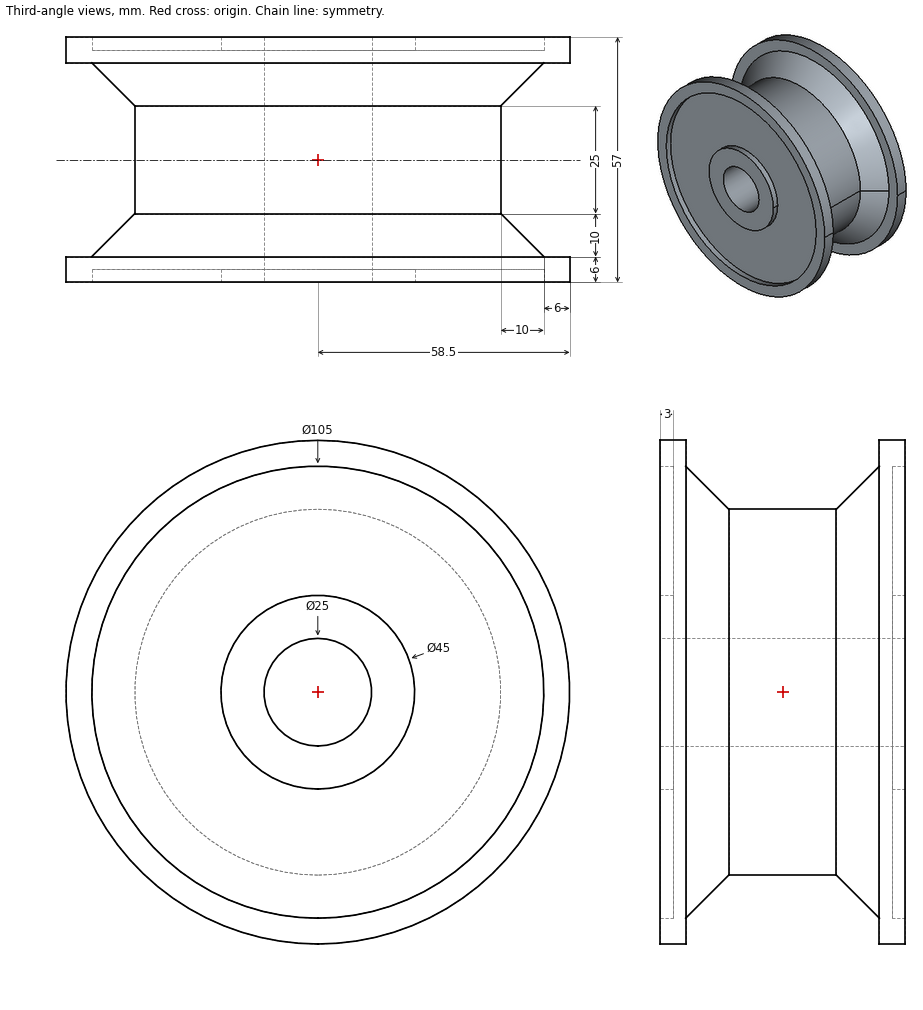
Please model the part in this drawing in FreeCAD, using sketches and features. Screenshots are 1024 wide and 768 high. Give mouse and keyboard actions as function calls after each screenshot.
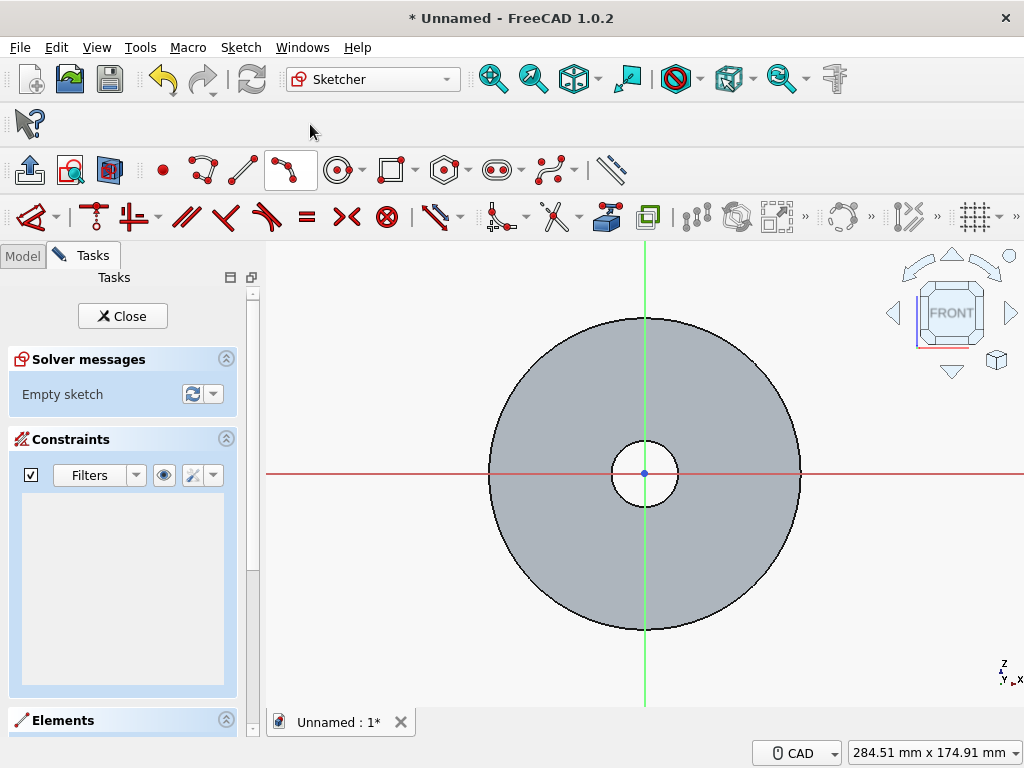
click(338, 170)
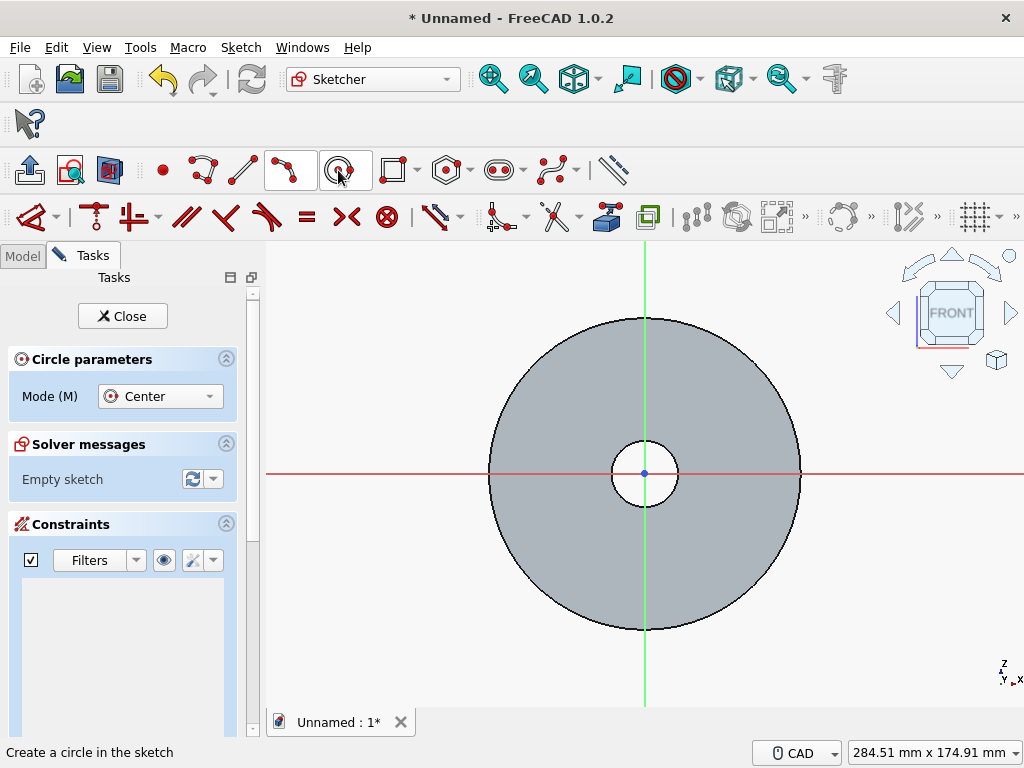
click(645, 474)
click(744, 375)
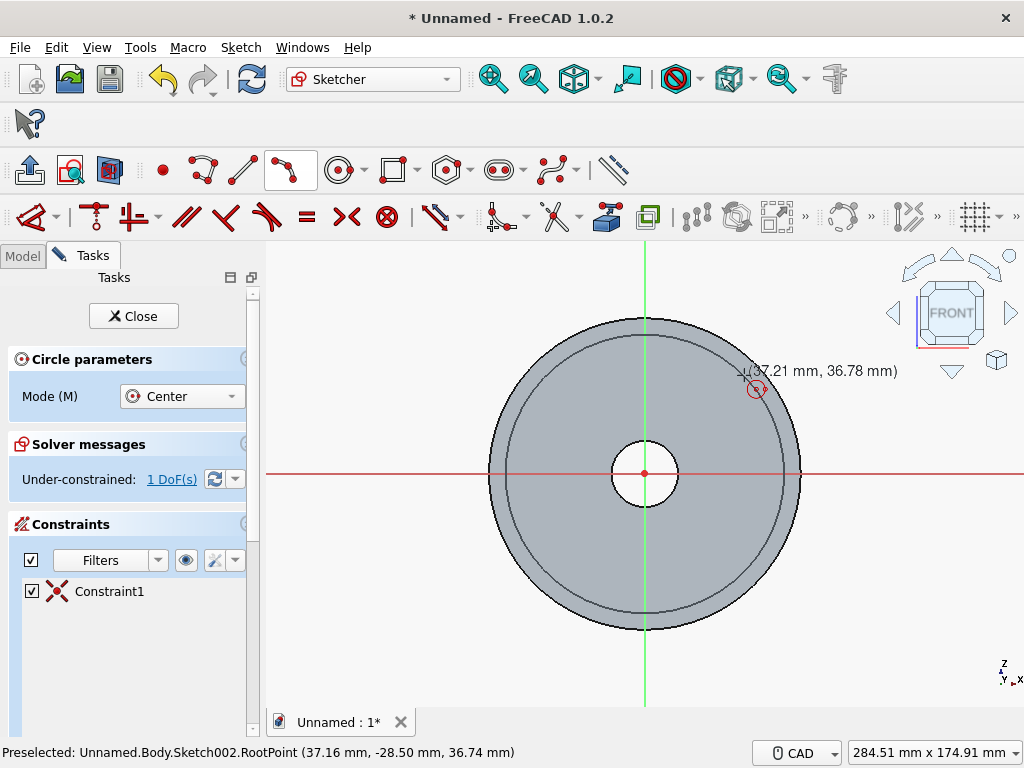
click(645, 474)
click(687, 432)
key(Escape)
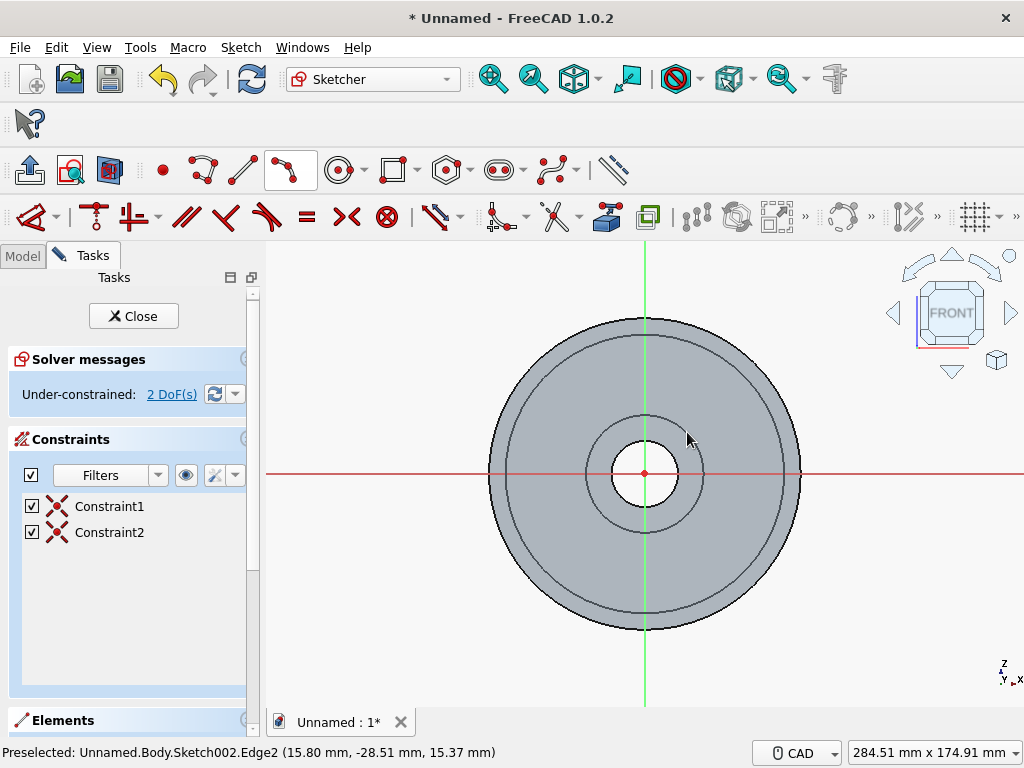
click(32, 218)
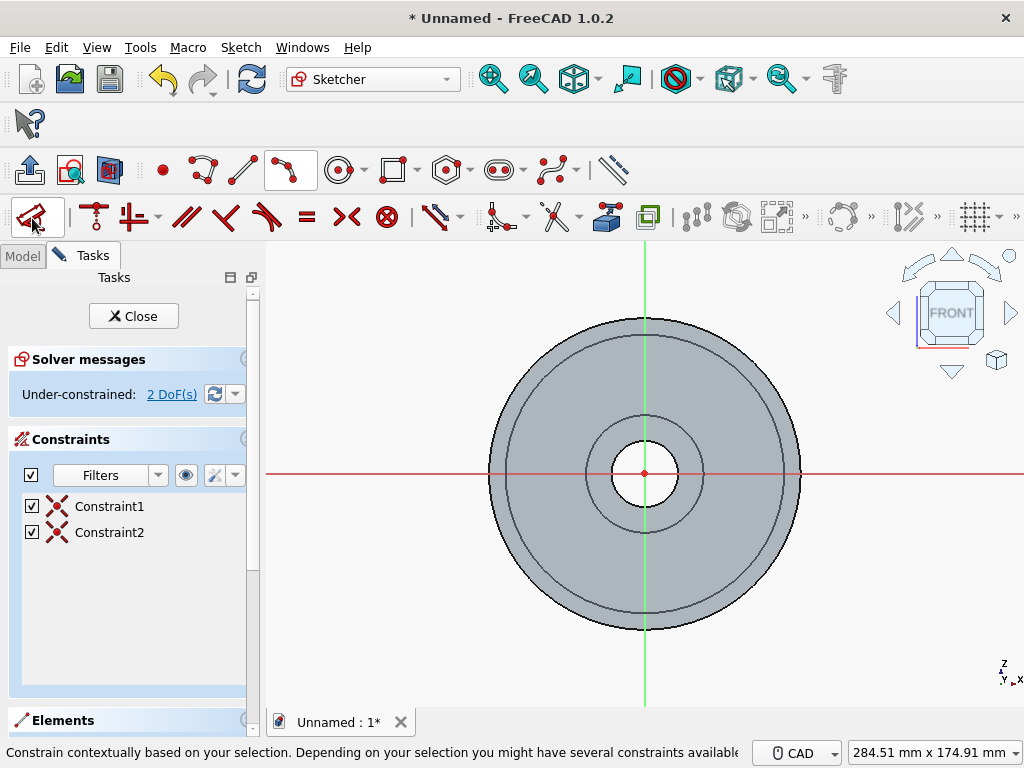
click(743, 375)
click(766, 352)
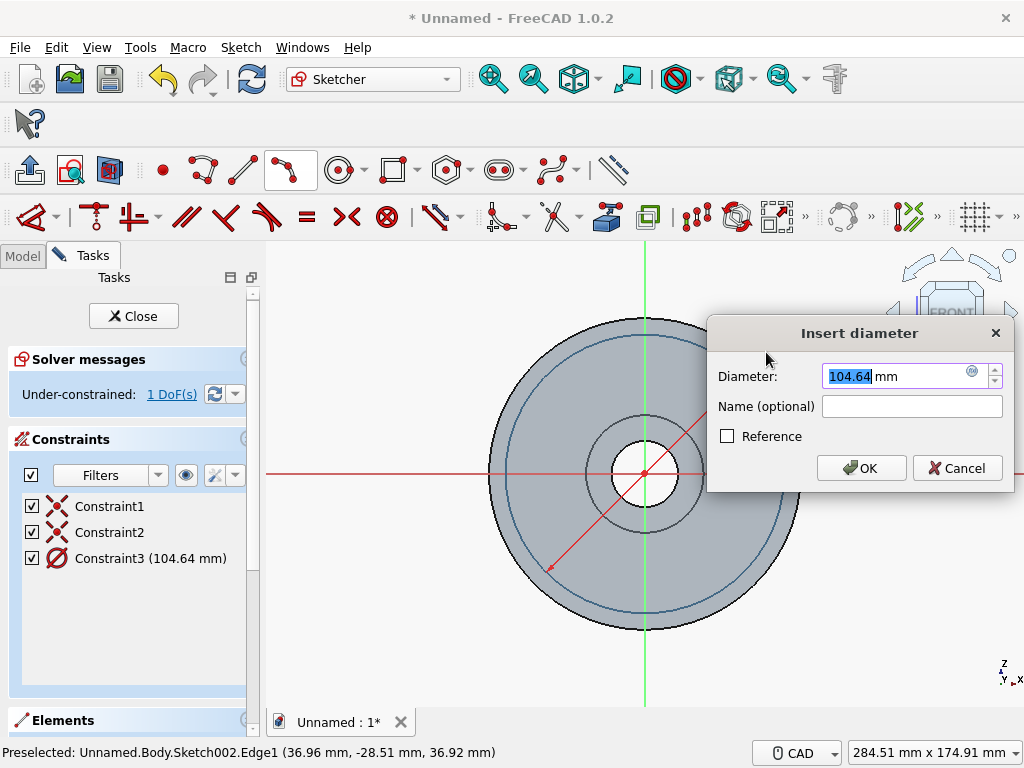
text(105)
key(Return)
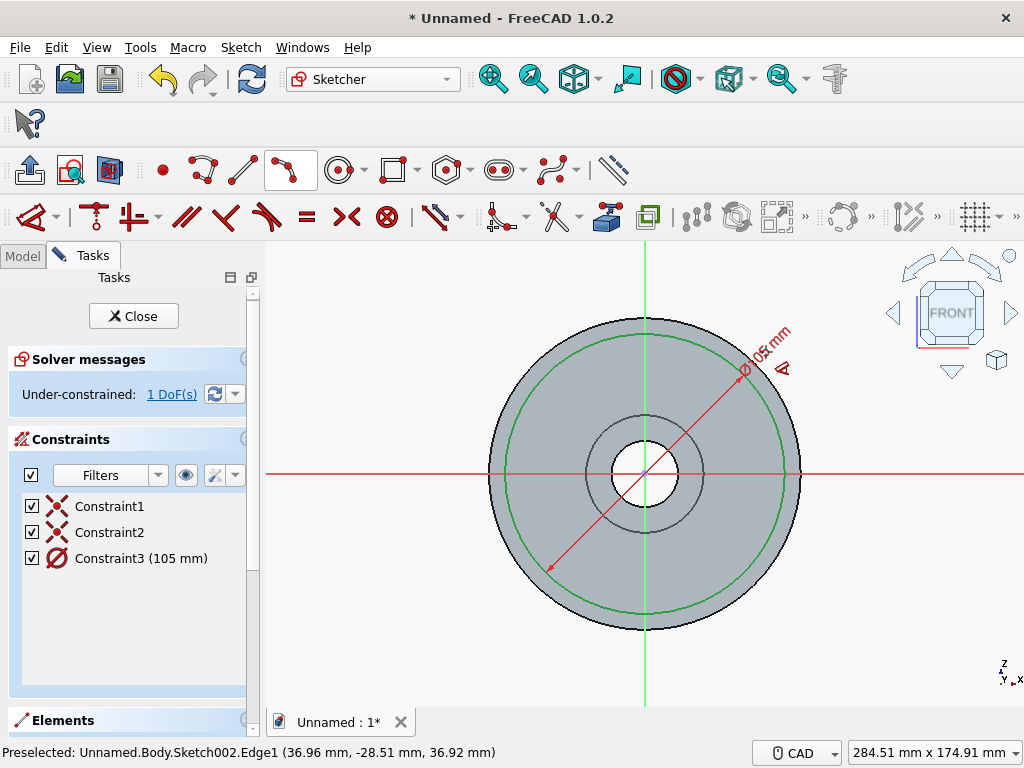
click(686, 432)
click(708, 409)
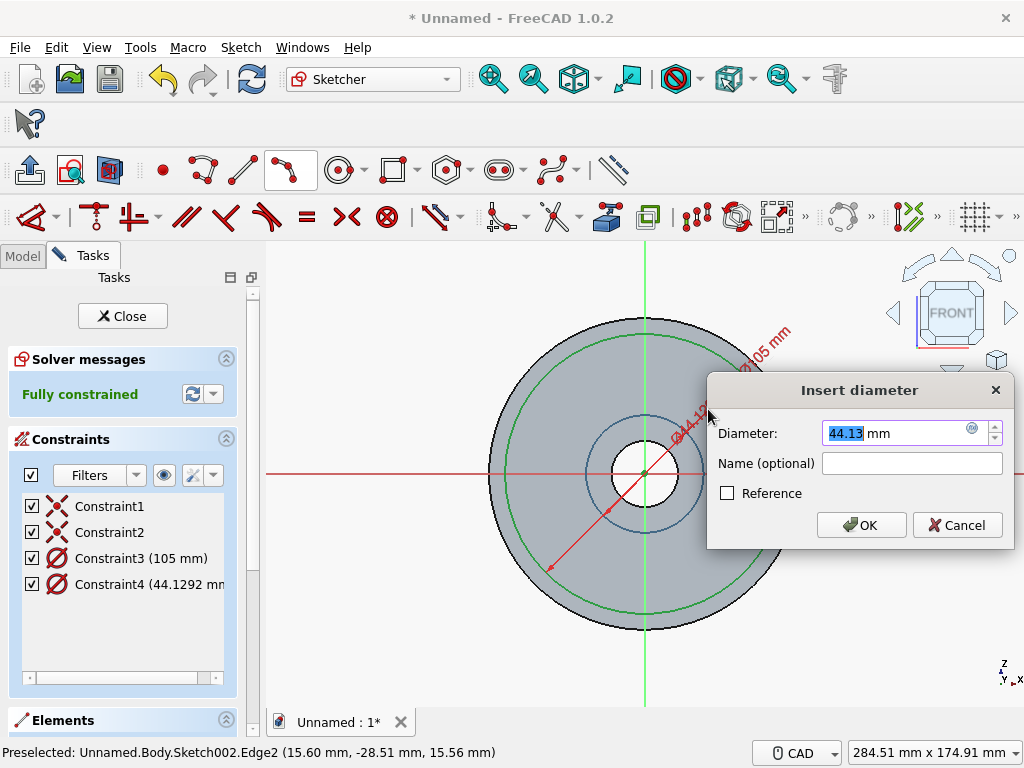
text(45)
key(Return)
key(Escape)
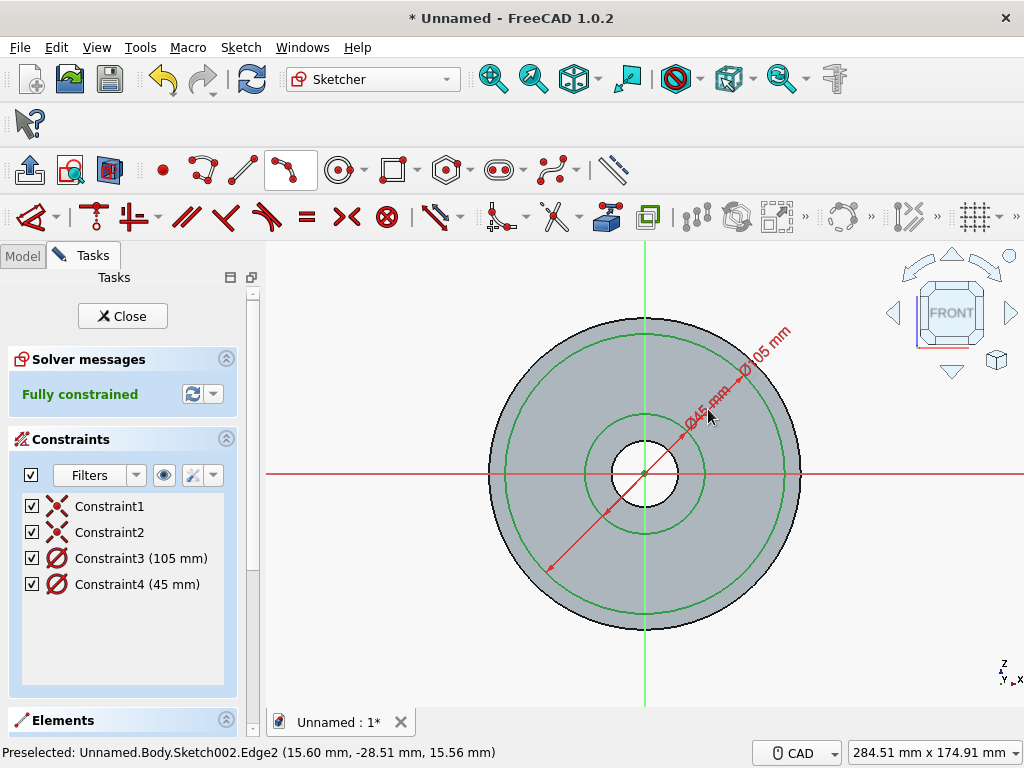
click(123, 316)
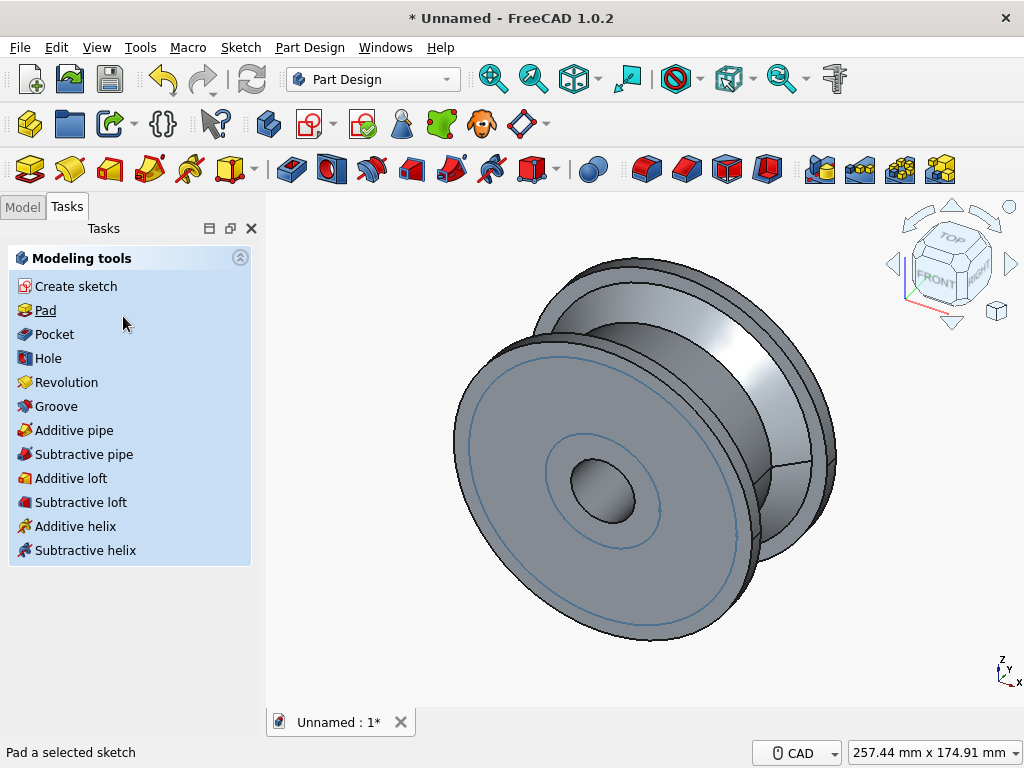
click(292, 170)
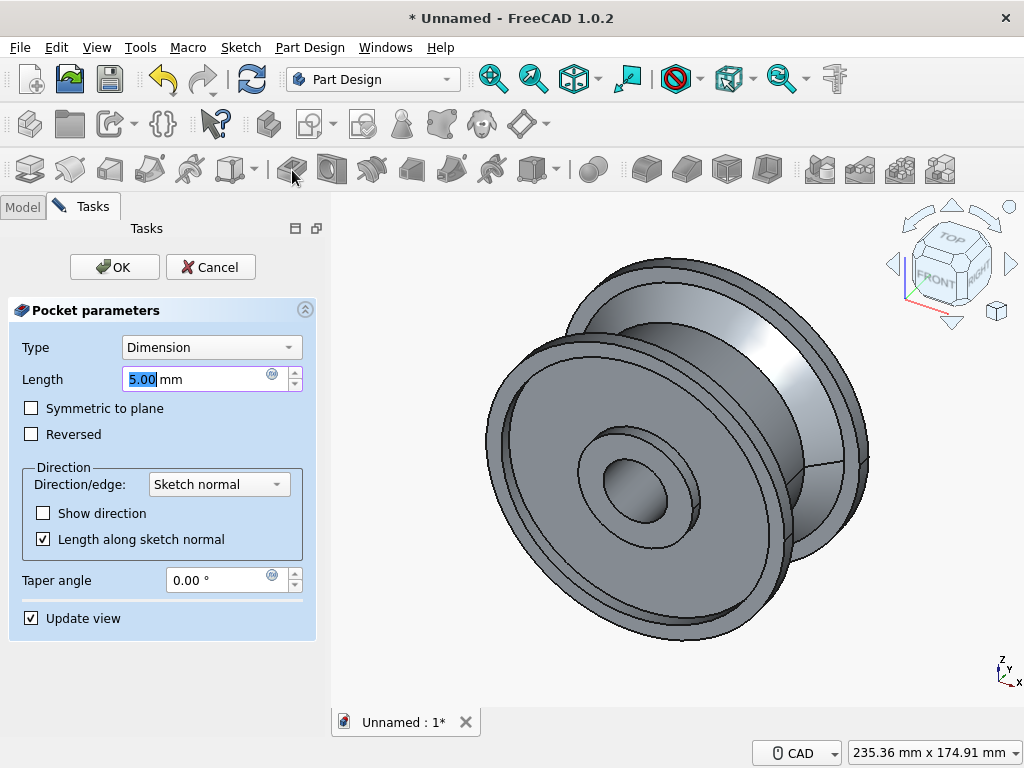
text(3)
key(Tab)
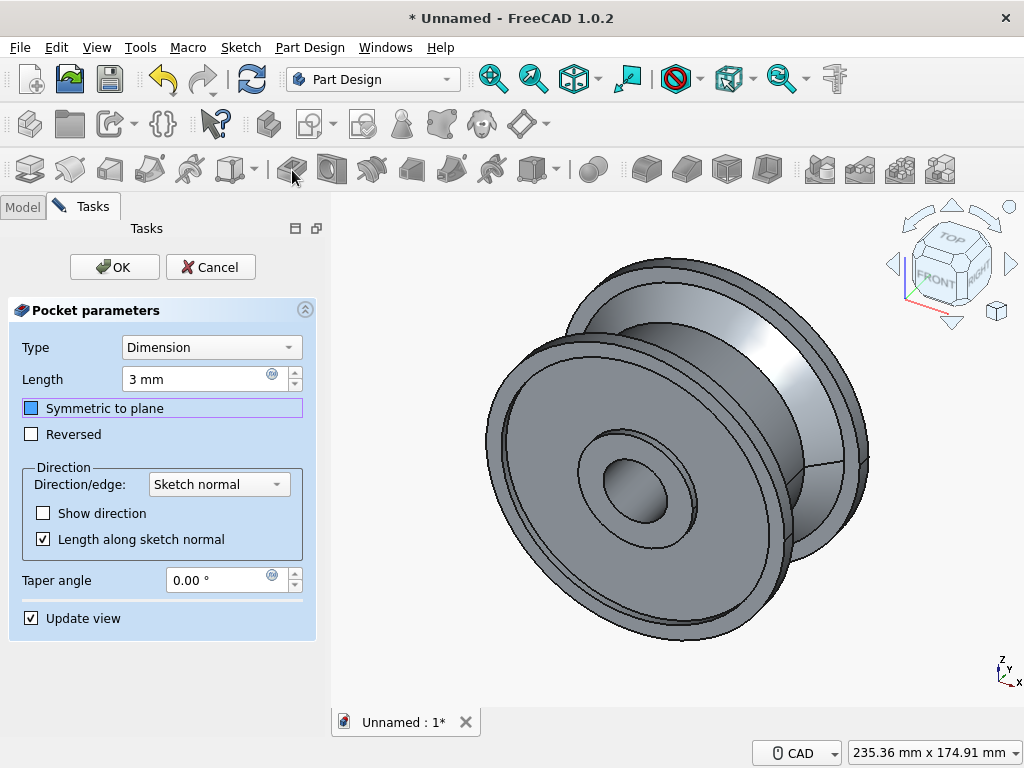
click(115, 267)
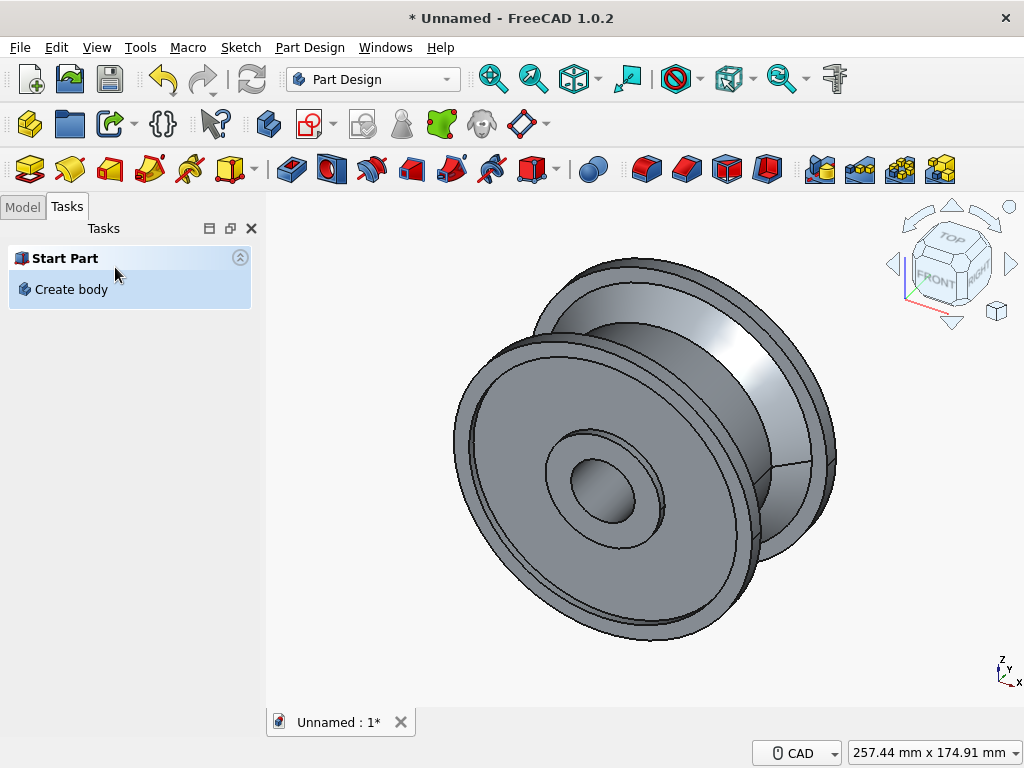
click(23, 206)